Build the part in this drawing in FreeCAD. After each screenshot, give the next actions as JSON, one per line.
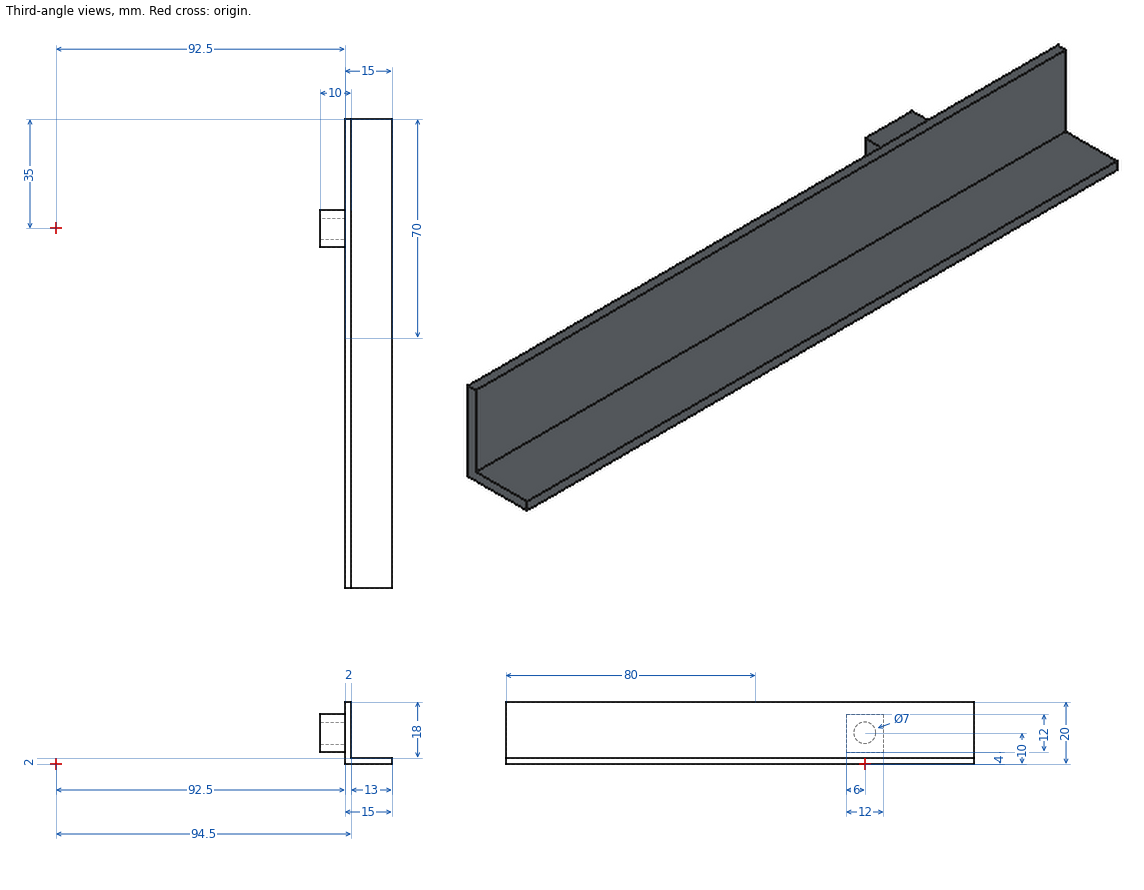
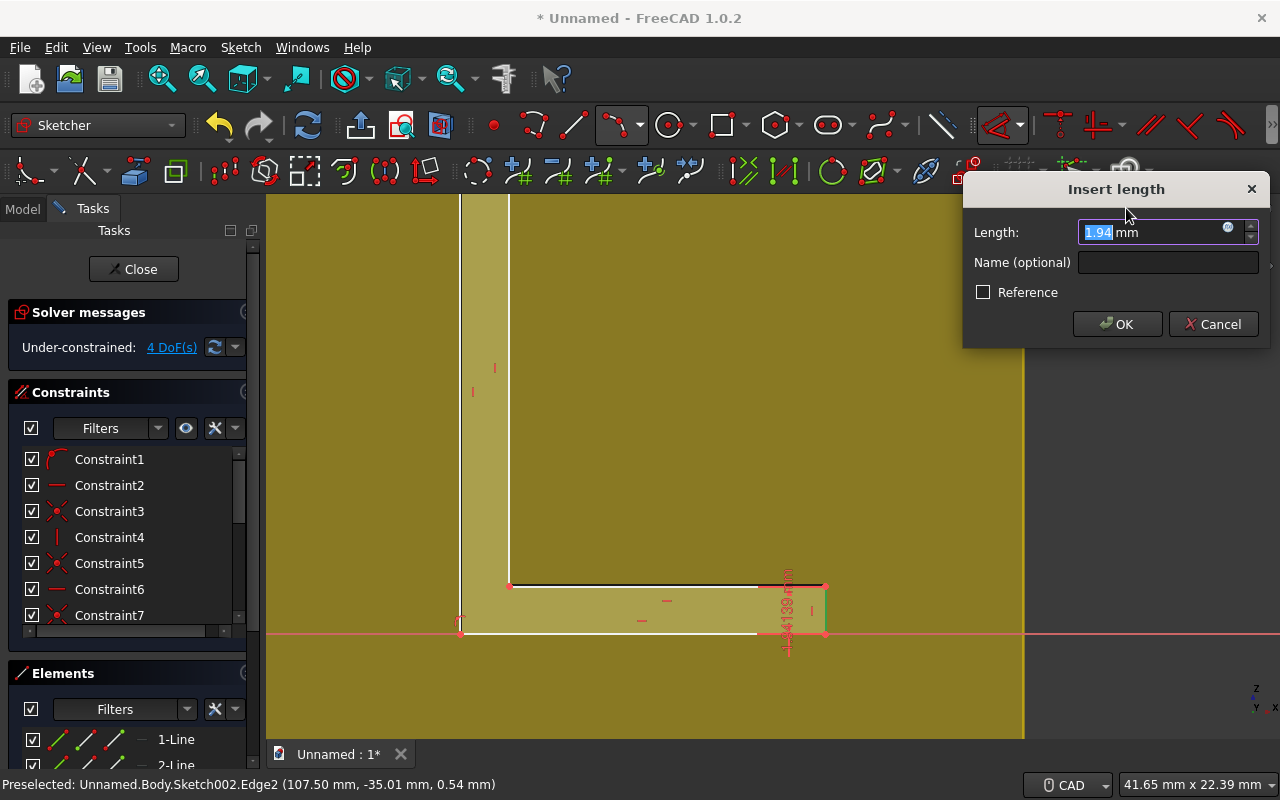
{"action": "type", "text": "2"}
{"action": "key", "text": "Return"}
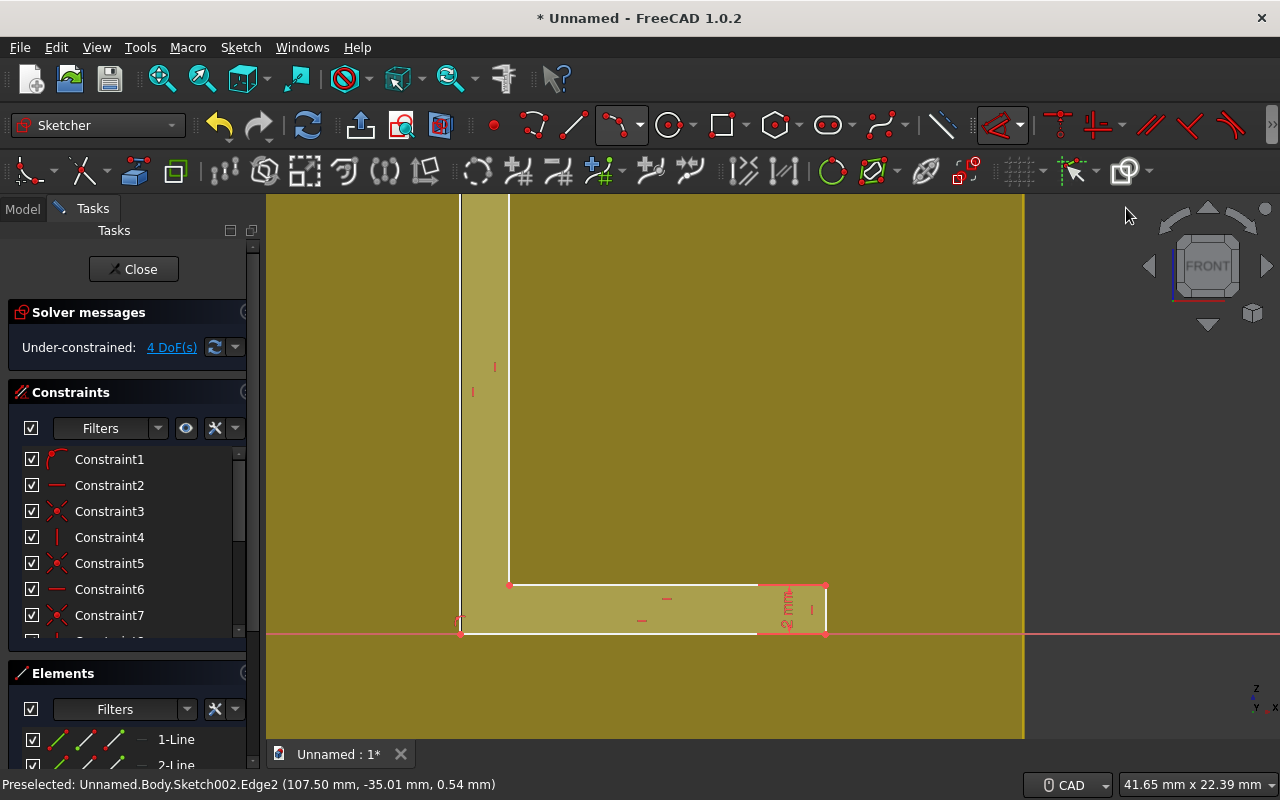
{"action": "scroll", "coordinate": [829, 621], "scroll_direction": "down", "scroll_amount": 2}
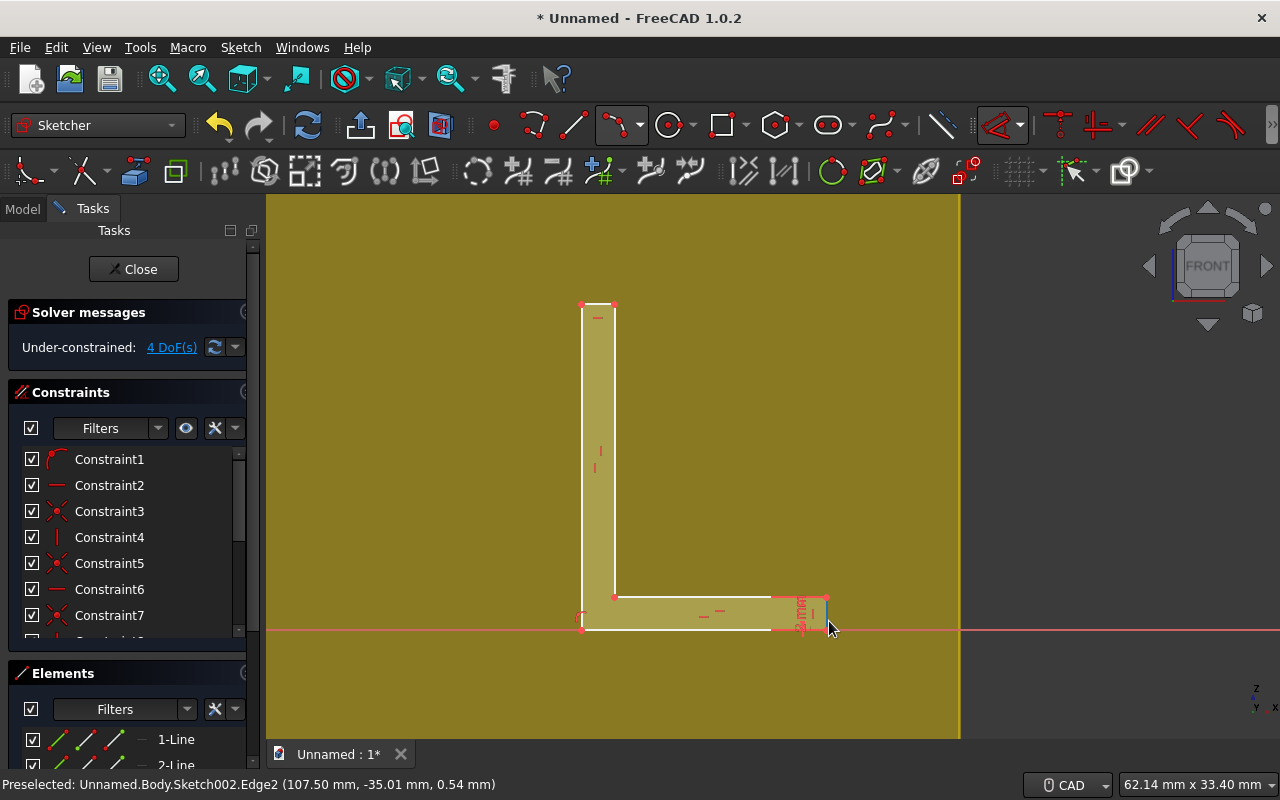
{"action": "scroll", "coordinate": [605, 304], "scroll_direction": "up", "scroll_amount": 2}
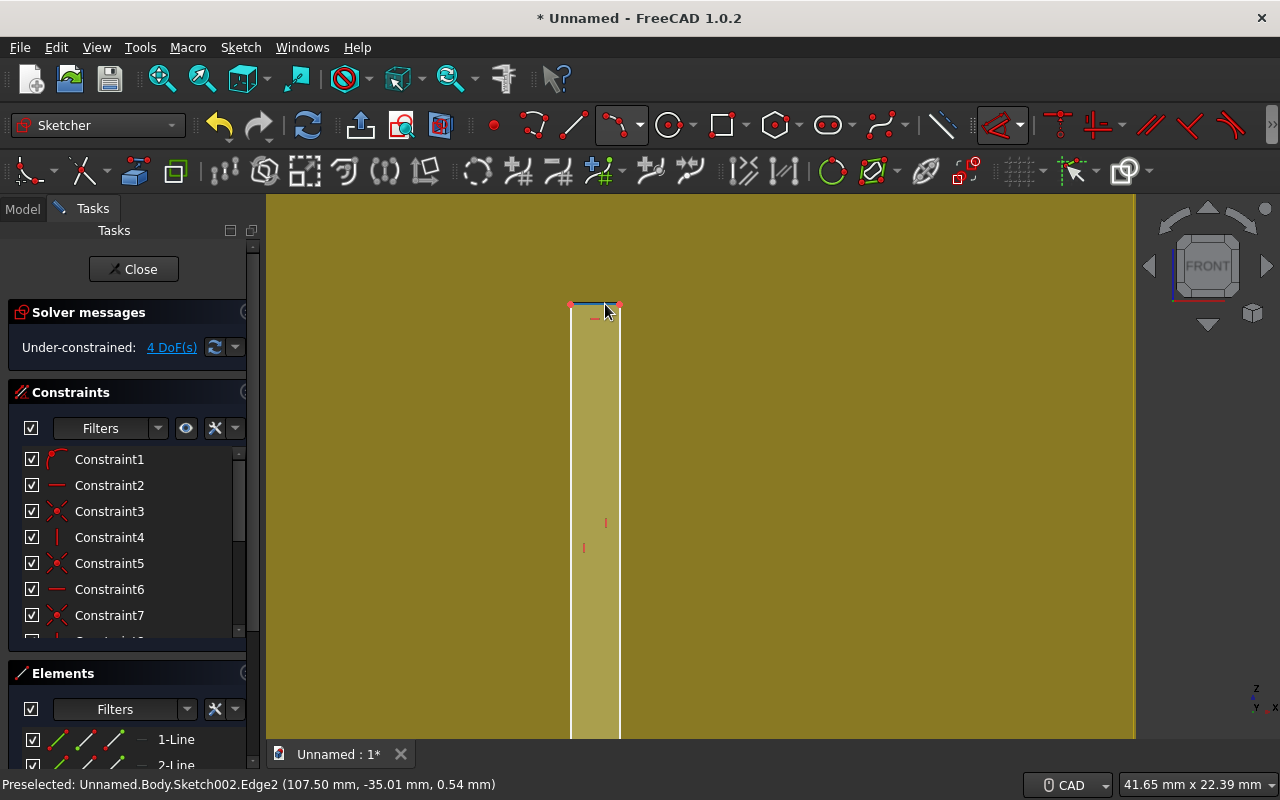
{"action": "left_click", "coordinate": [605, 304]}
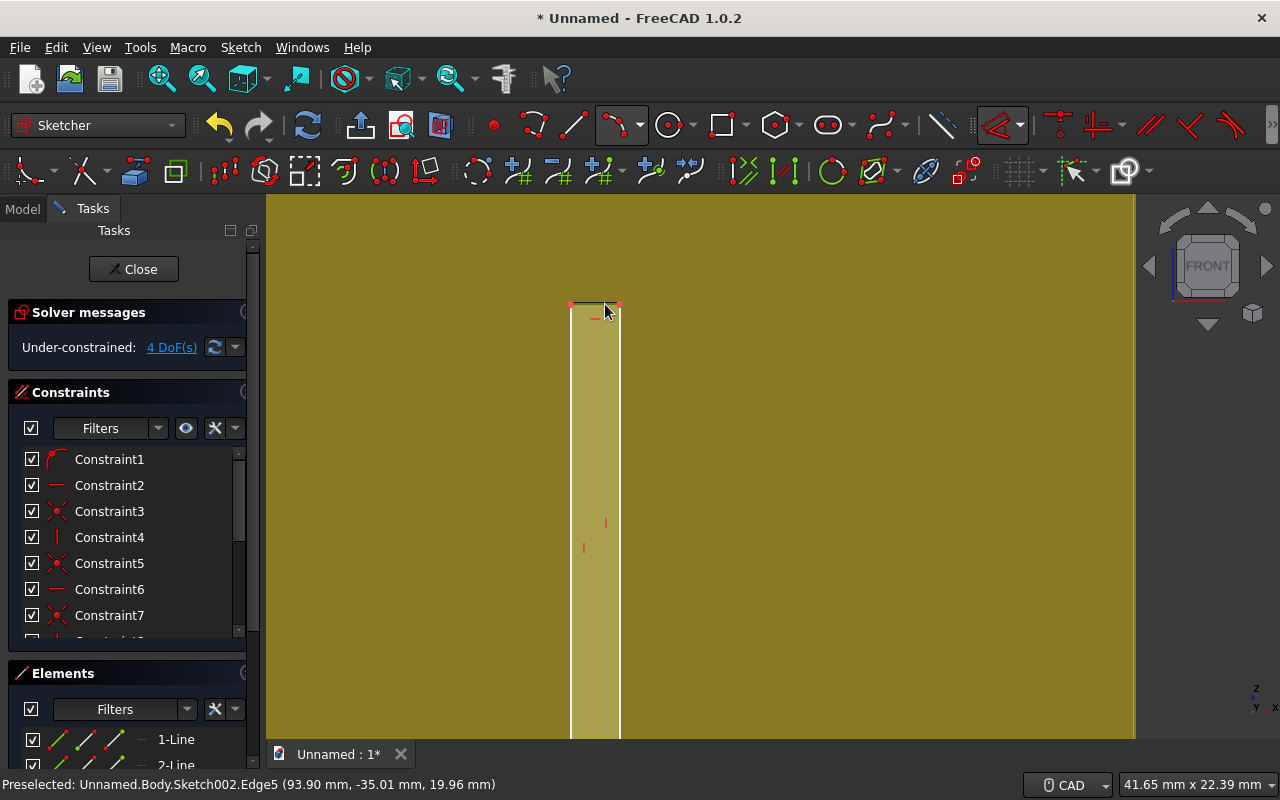
{"action": "key", "text": "l"}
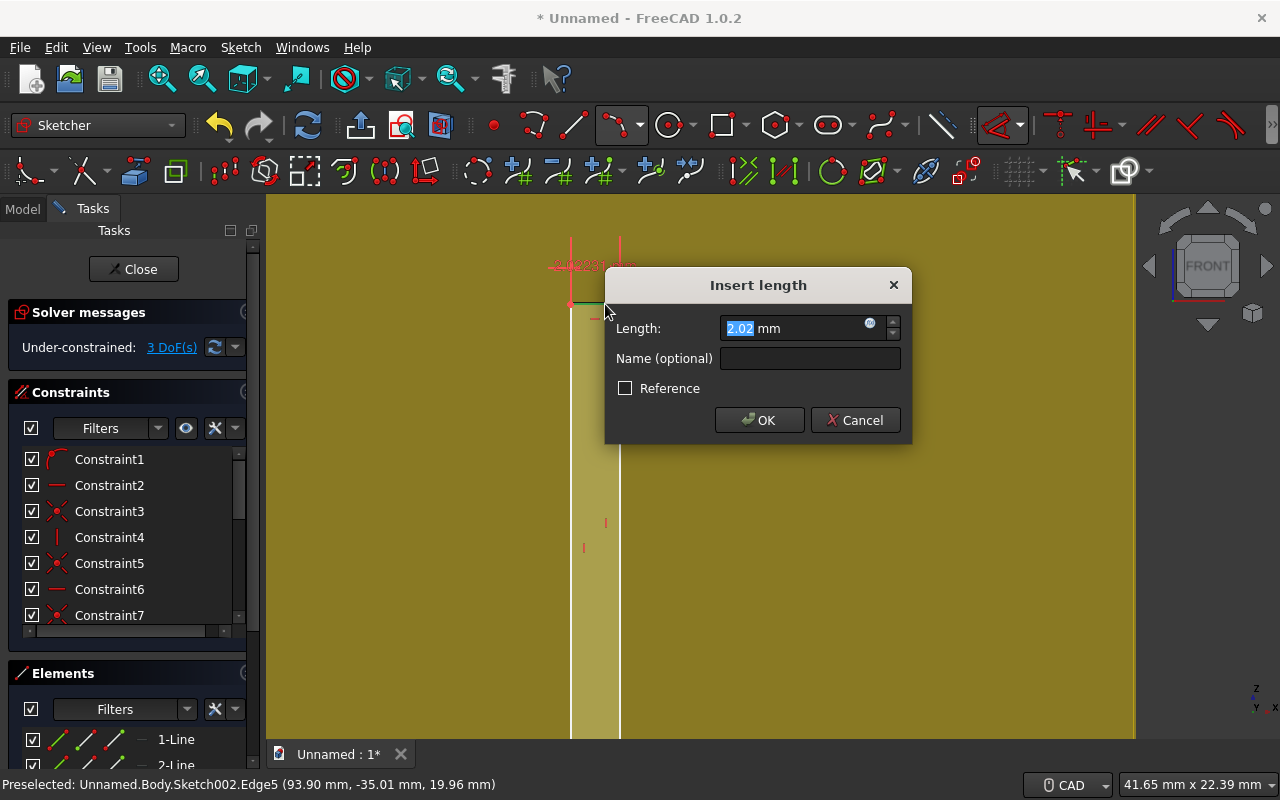
{"action": "type", "text": "2"}
{"action": "key", "text": "Return"}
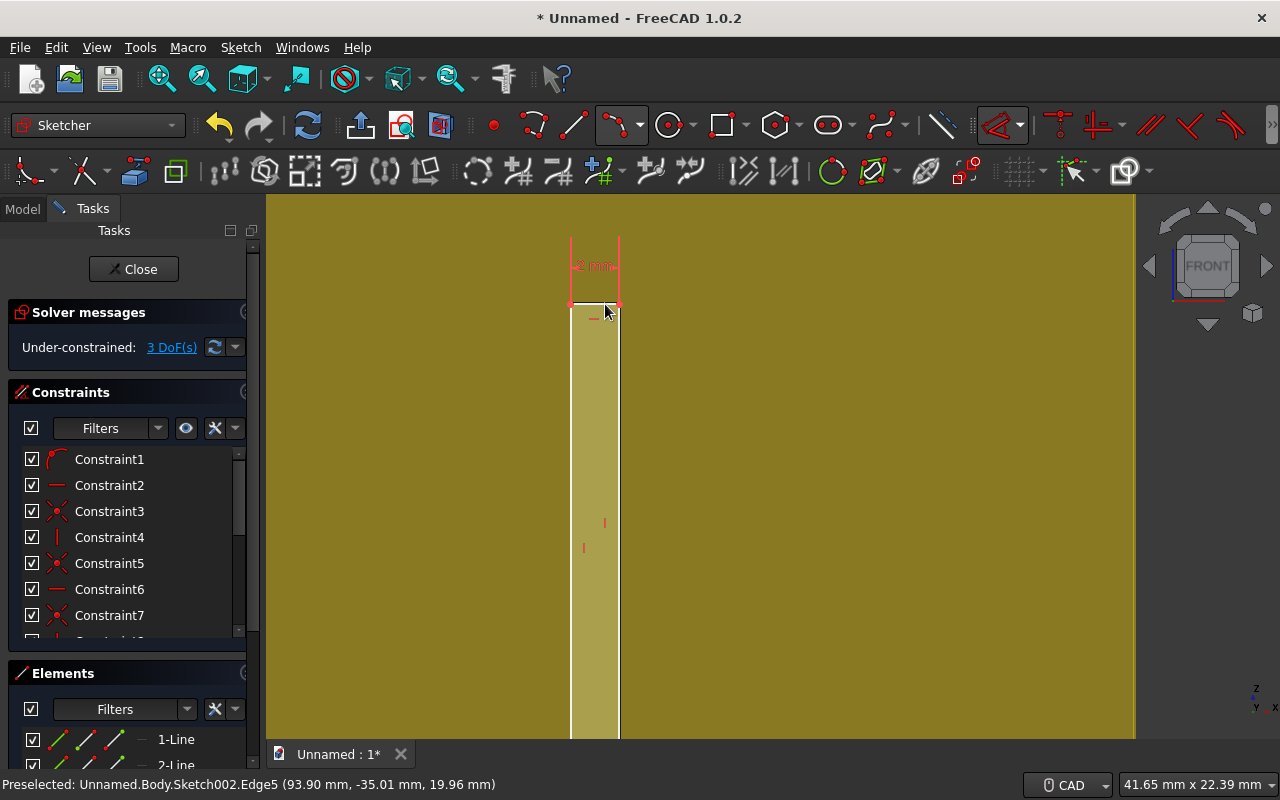
{"action": "scroll", "coordinate": [605, 303], "scroll_direction": "down", "scroll_amount": 2}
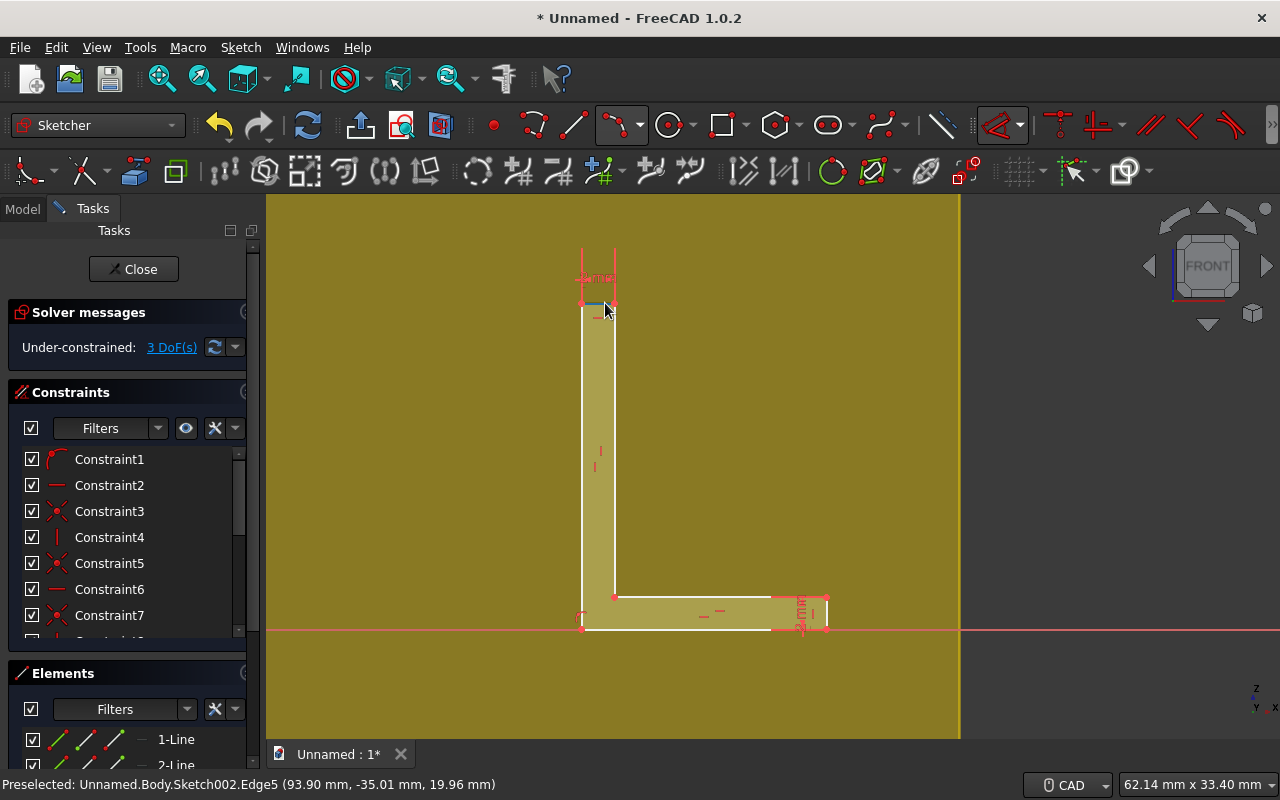
{"action": "left_click", "coordinate": [655, 630]}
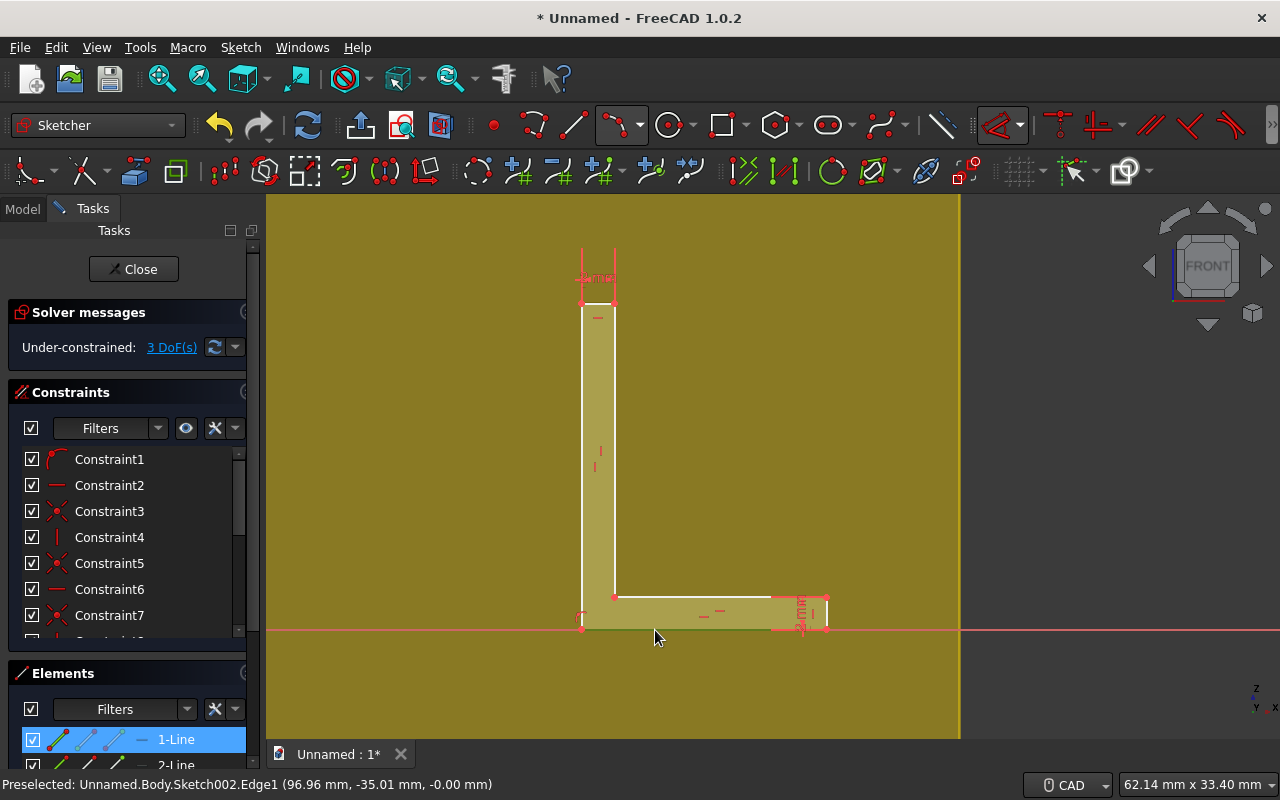
{"action": "left_click", "coordinate": [1022, 126]}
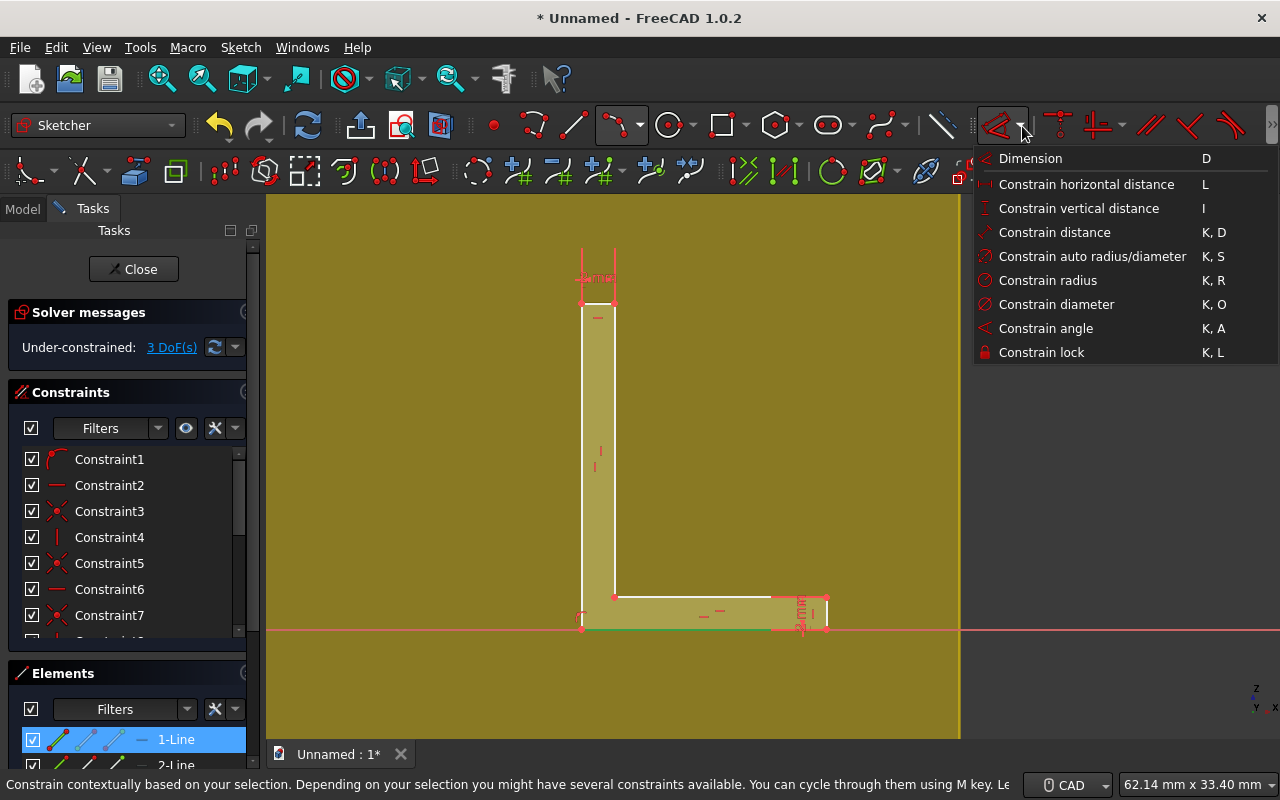
{"action": "left_click", "coordinate": [1126, 184]}